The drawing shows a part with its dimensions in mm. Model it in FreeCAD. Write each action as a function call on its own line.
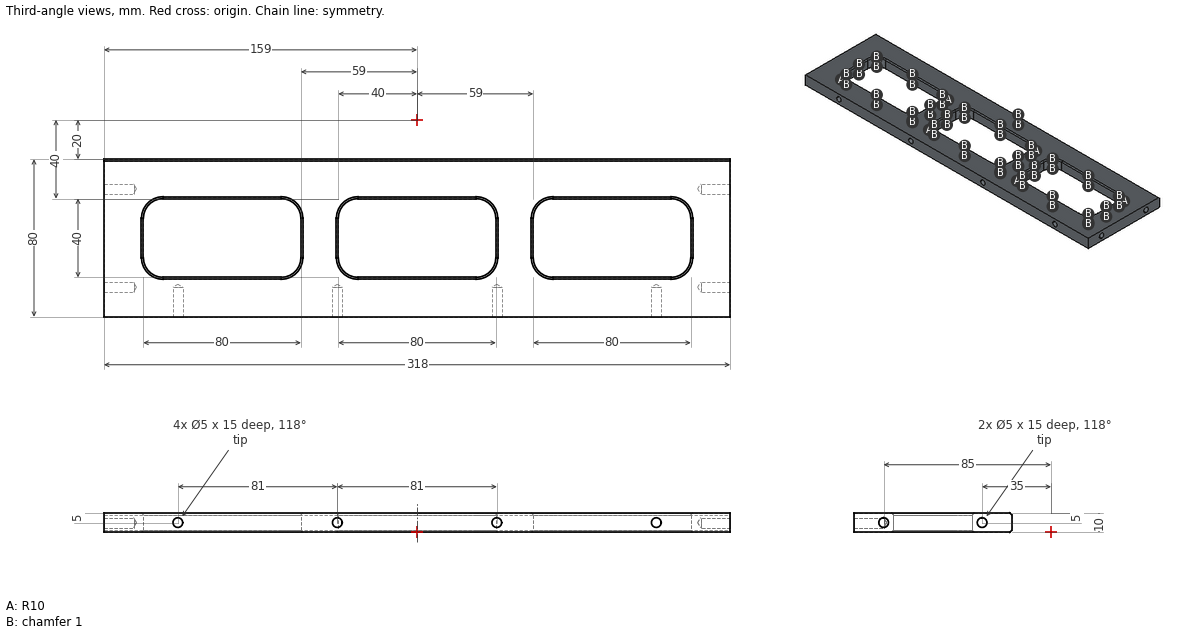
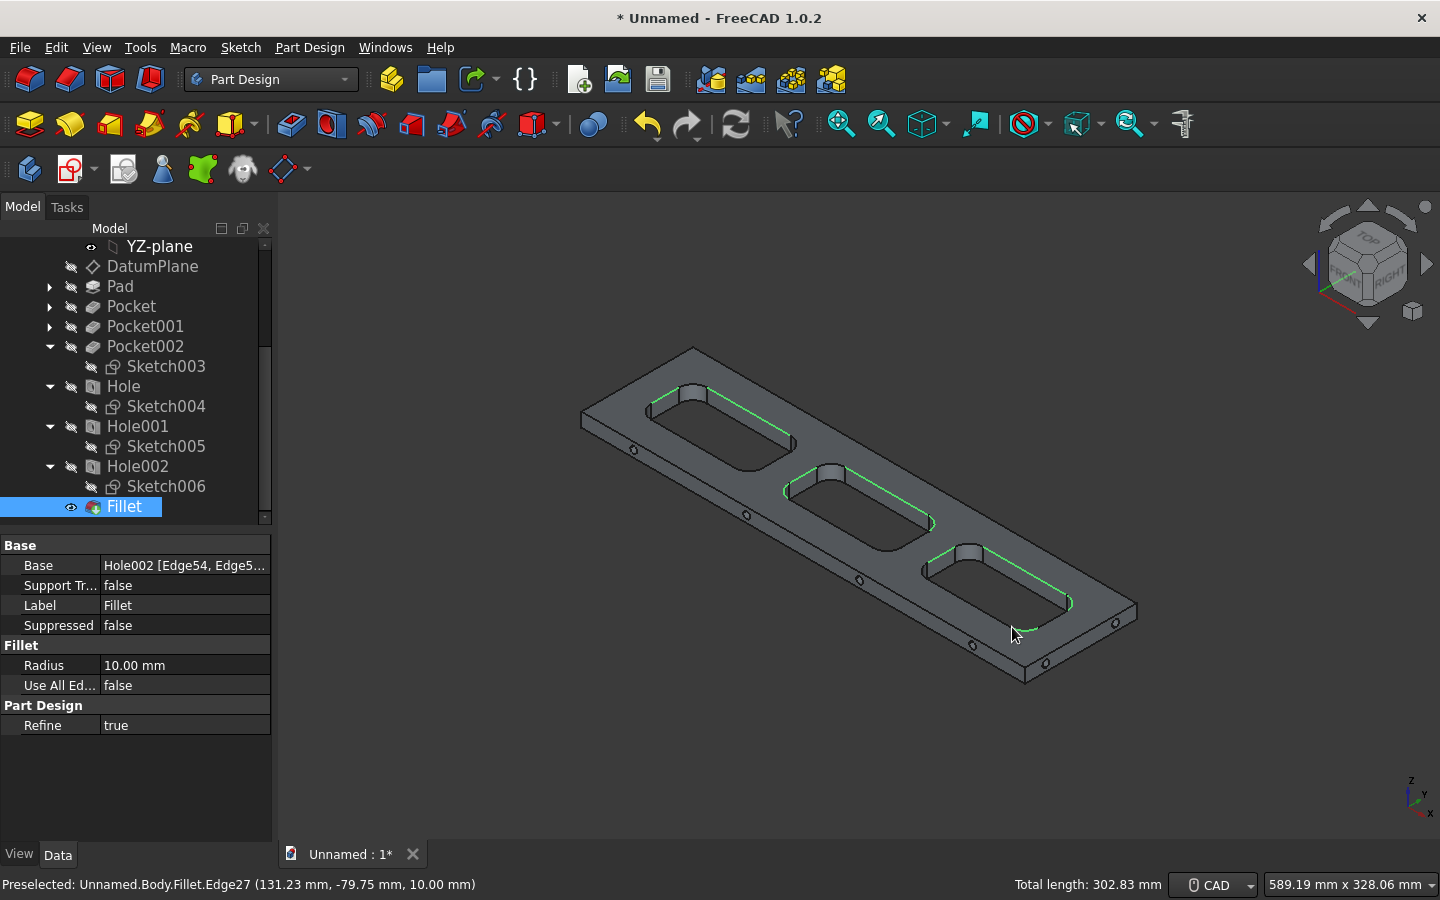
click(693, 383, ctrl)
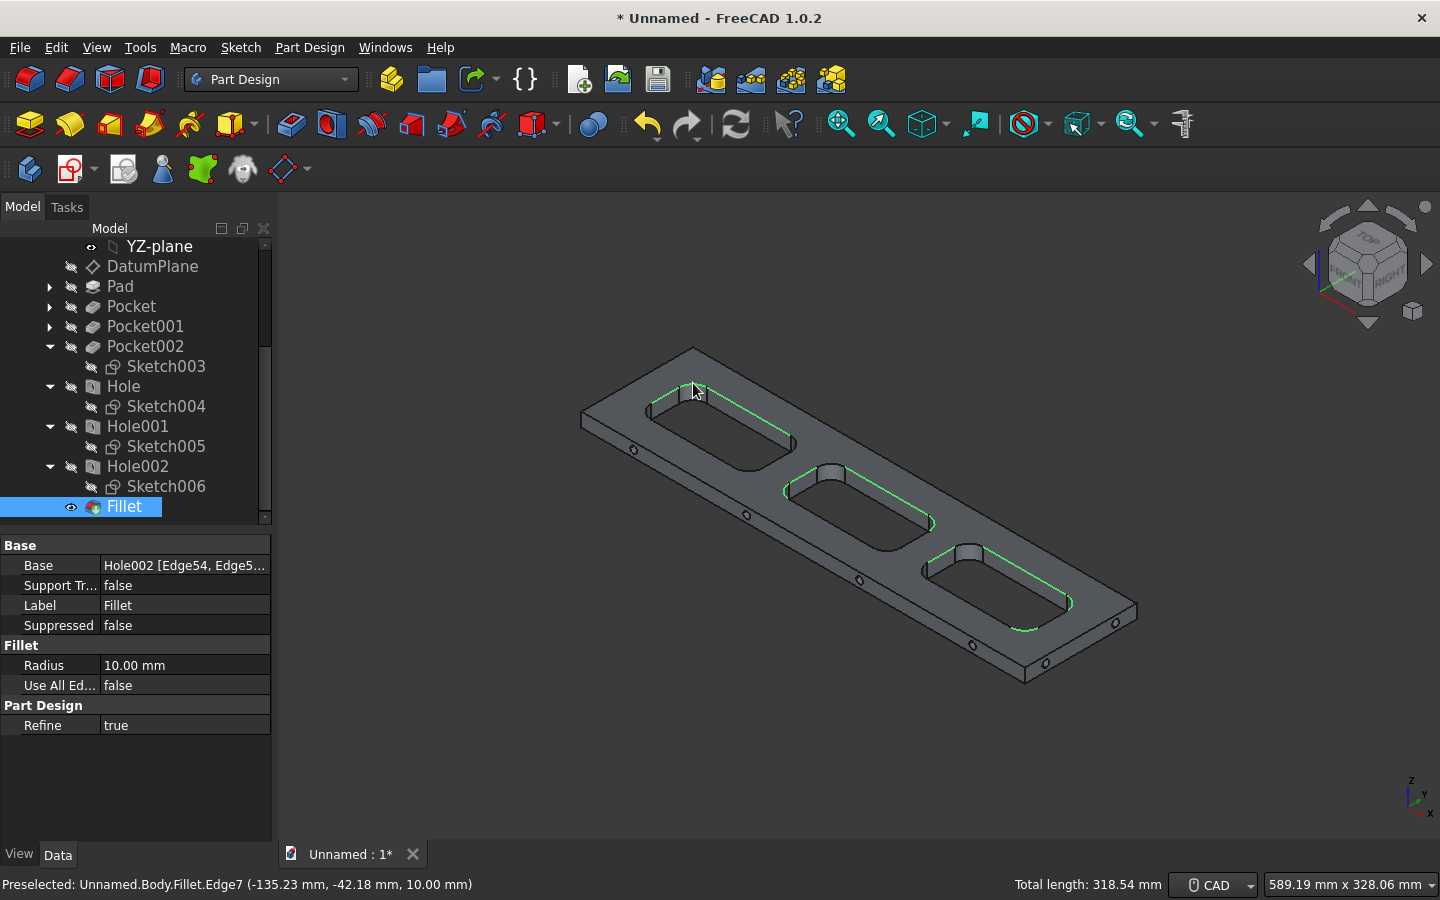
click(969, 543, ctrl)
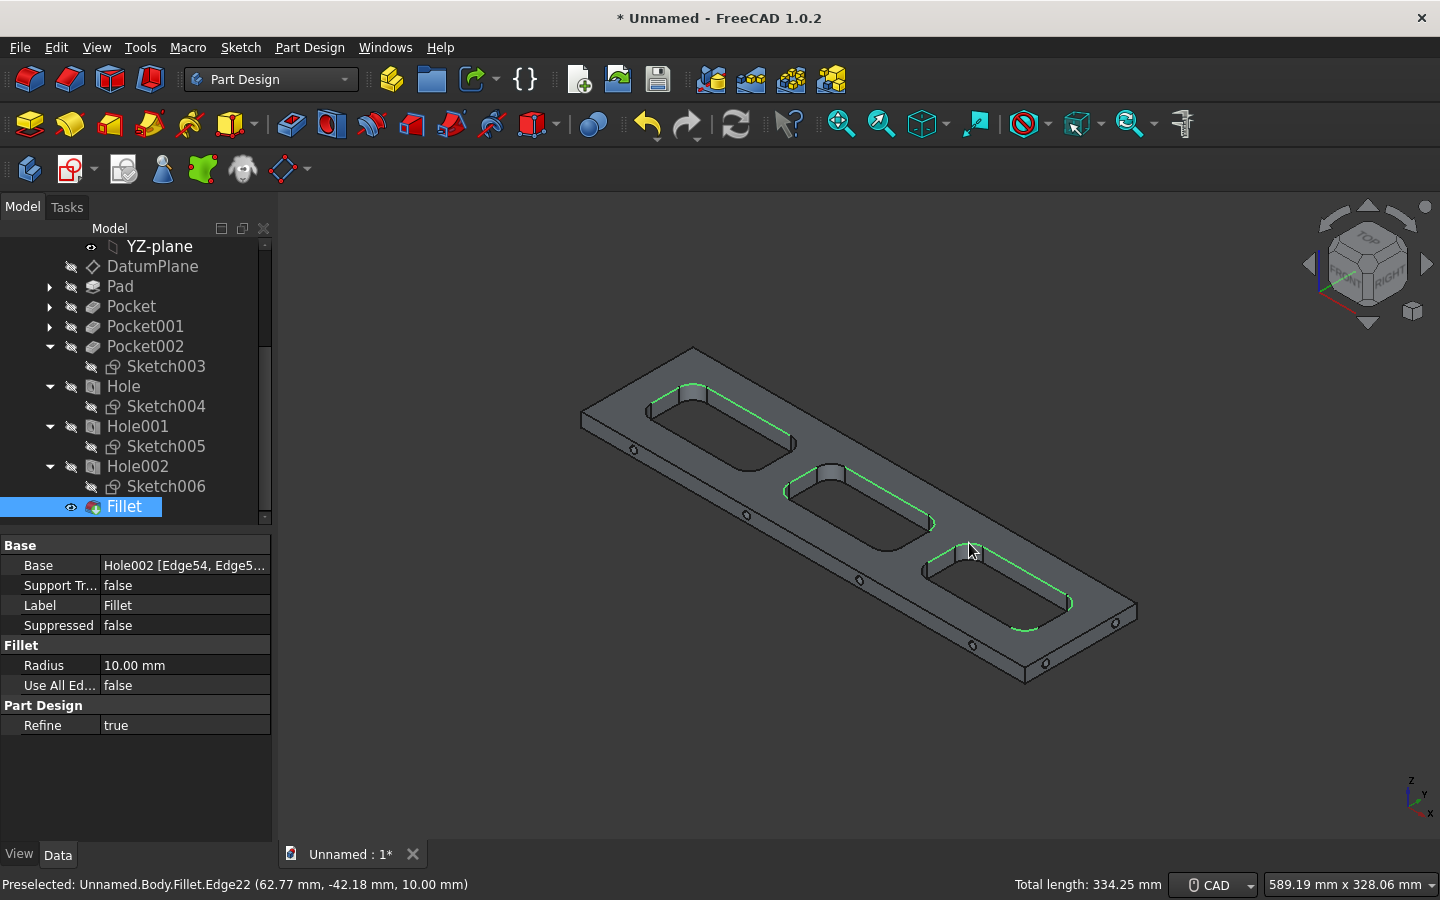
click(874, 547, ctrl)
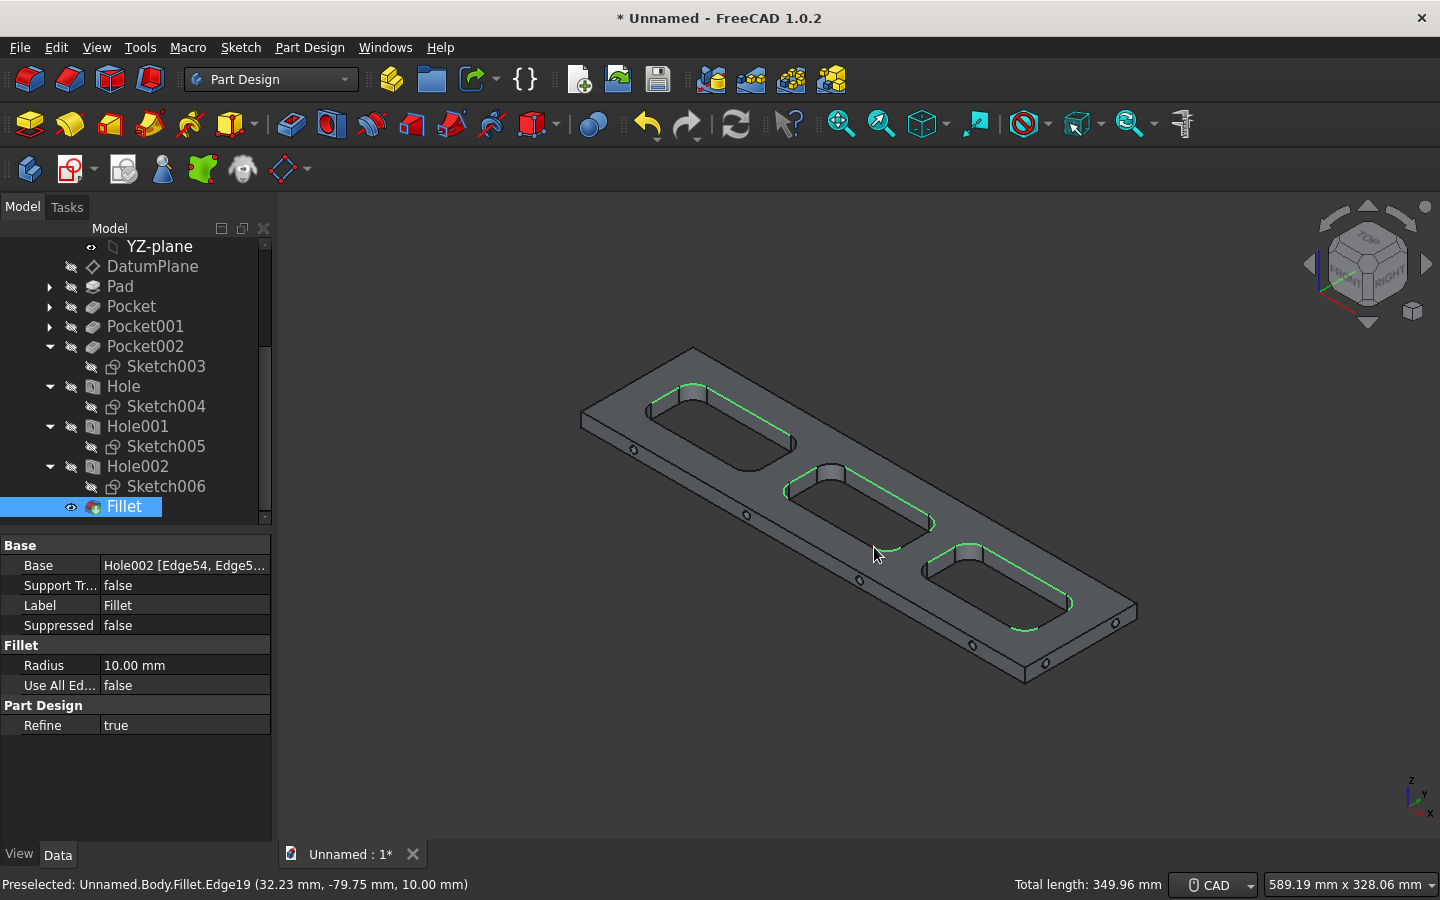
click(796, 443, ctrl)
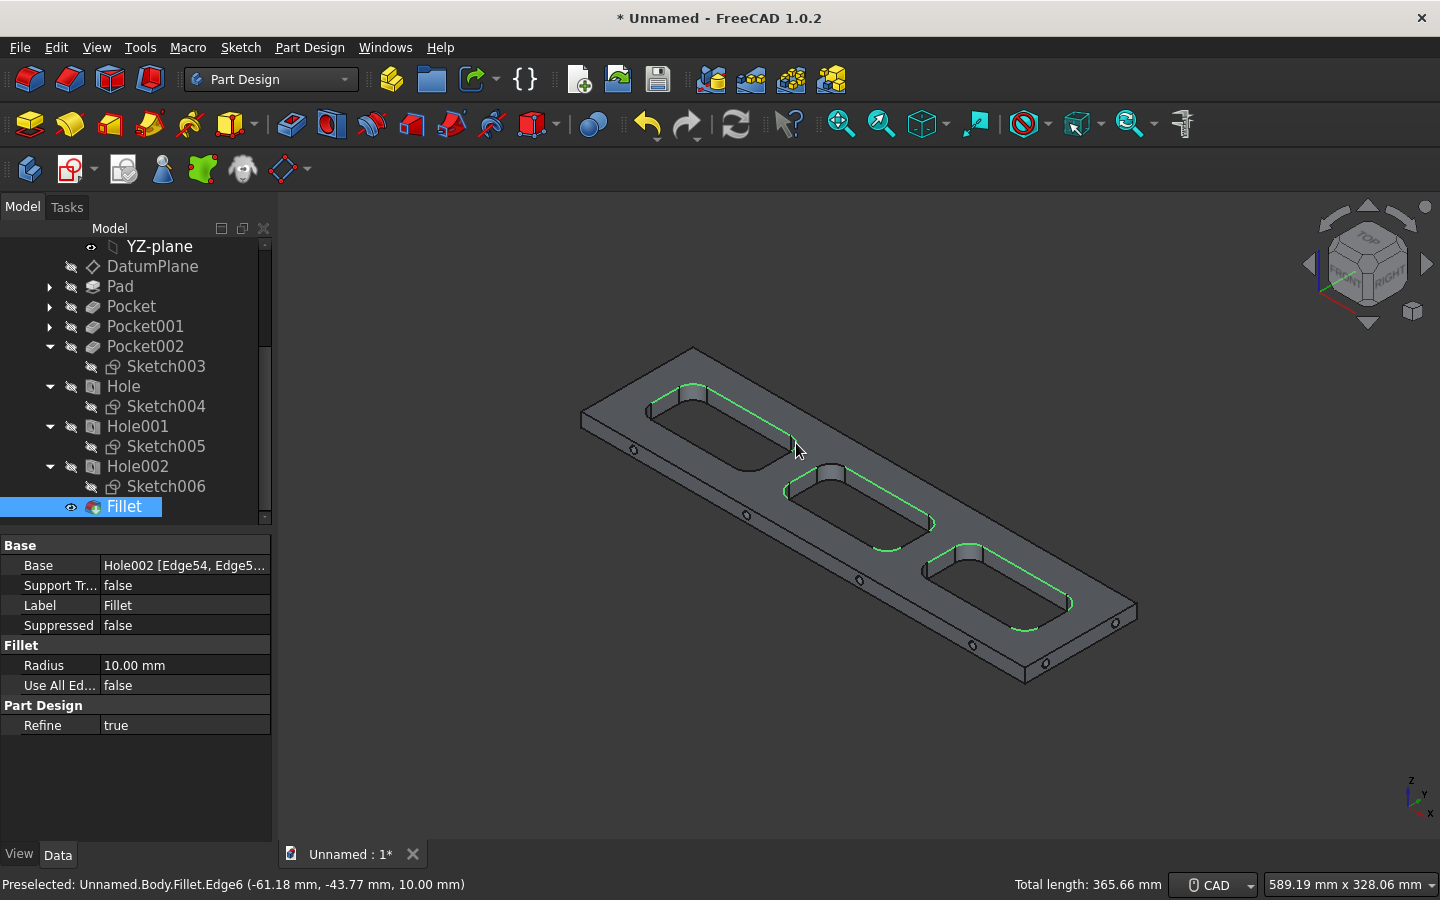
click(831, 463, ctrl)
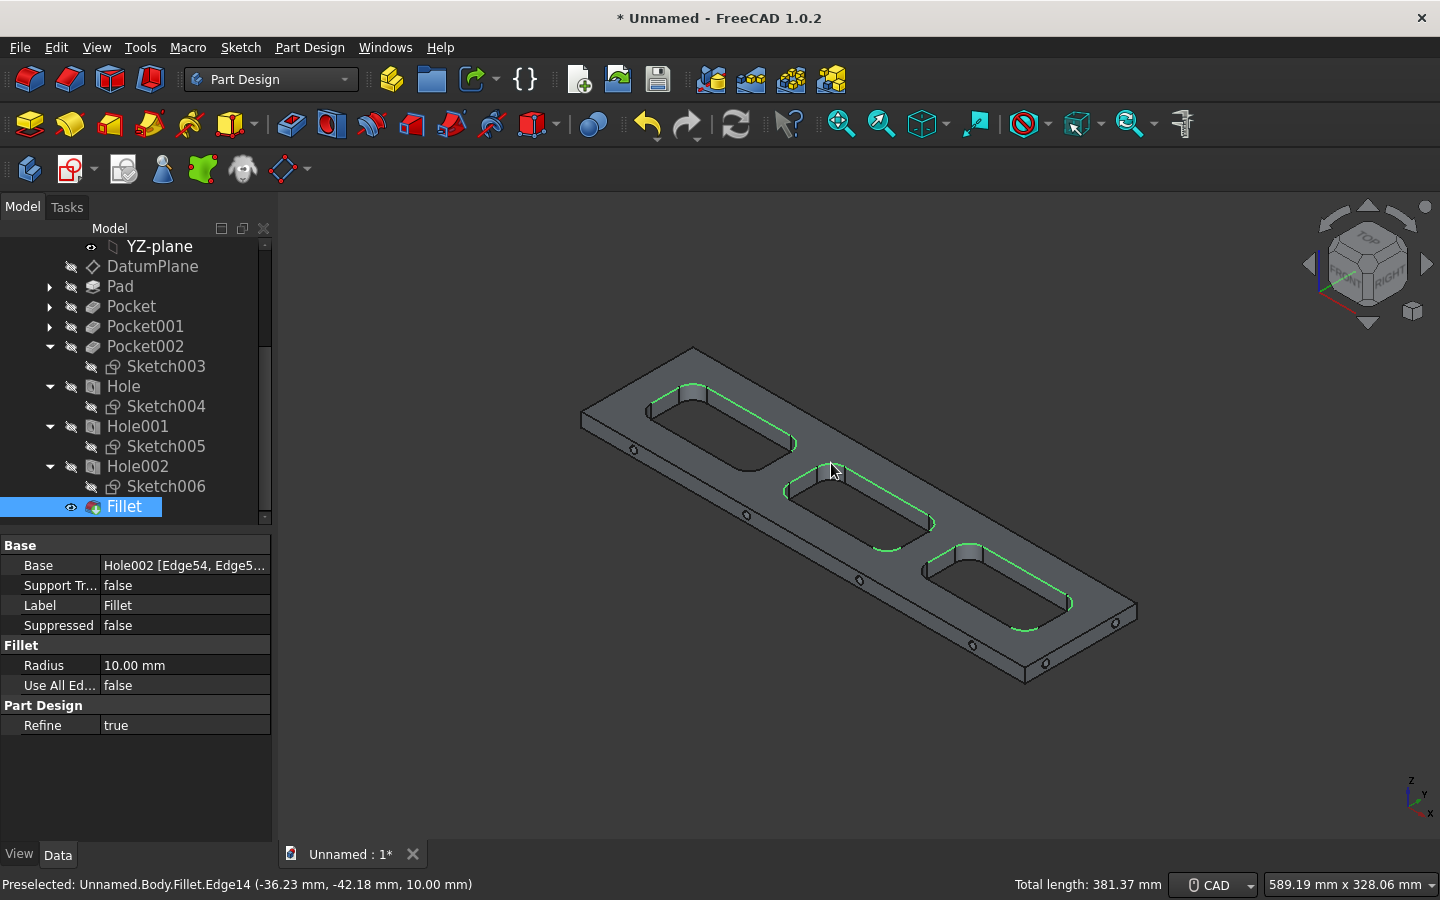
click(837, 480, ctrl)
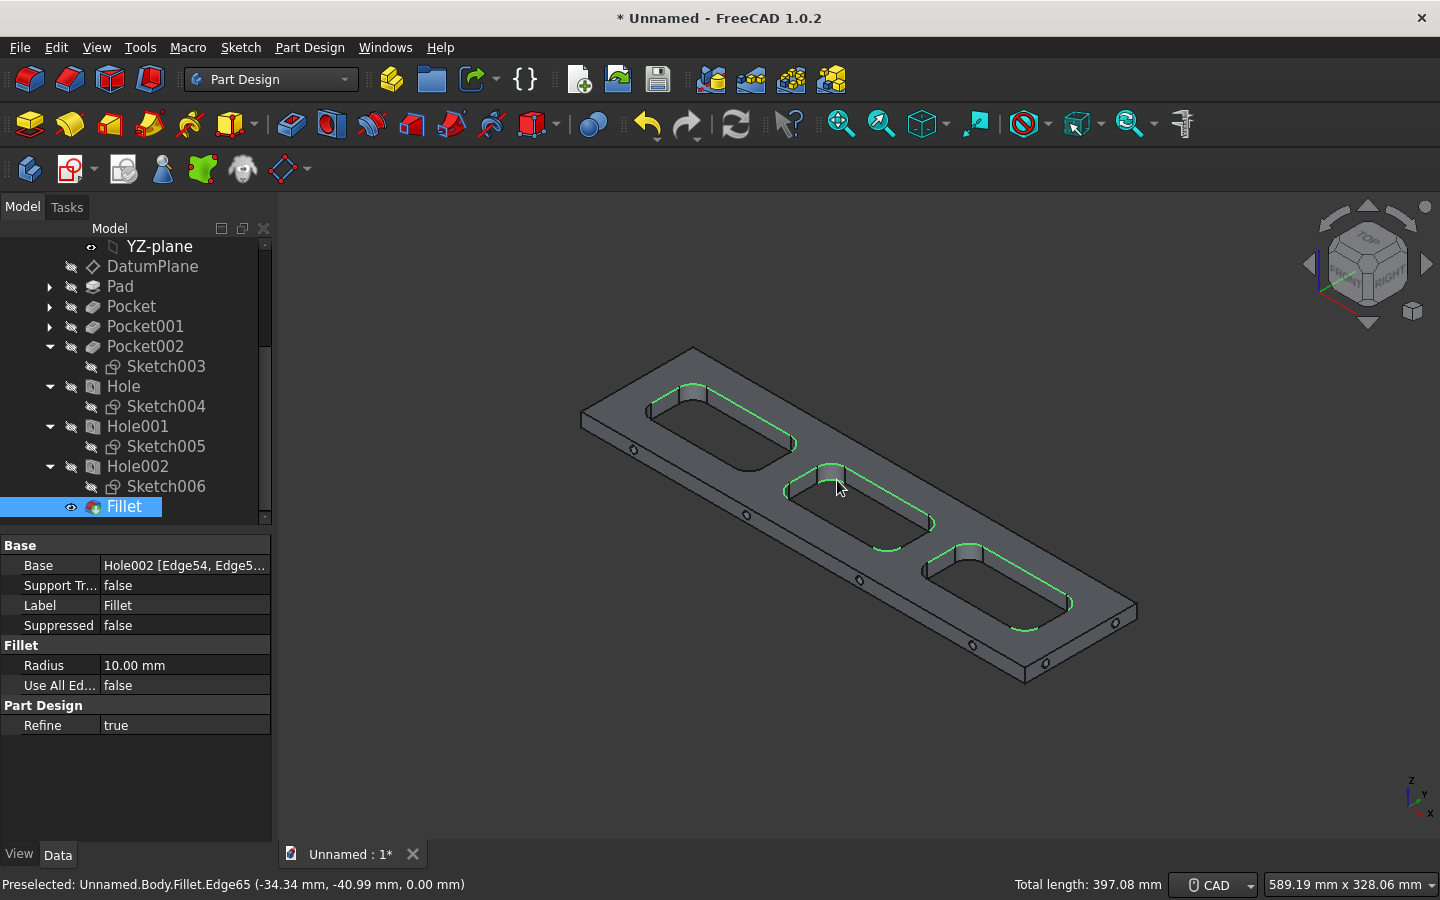
click(736, 467, ctrl)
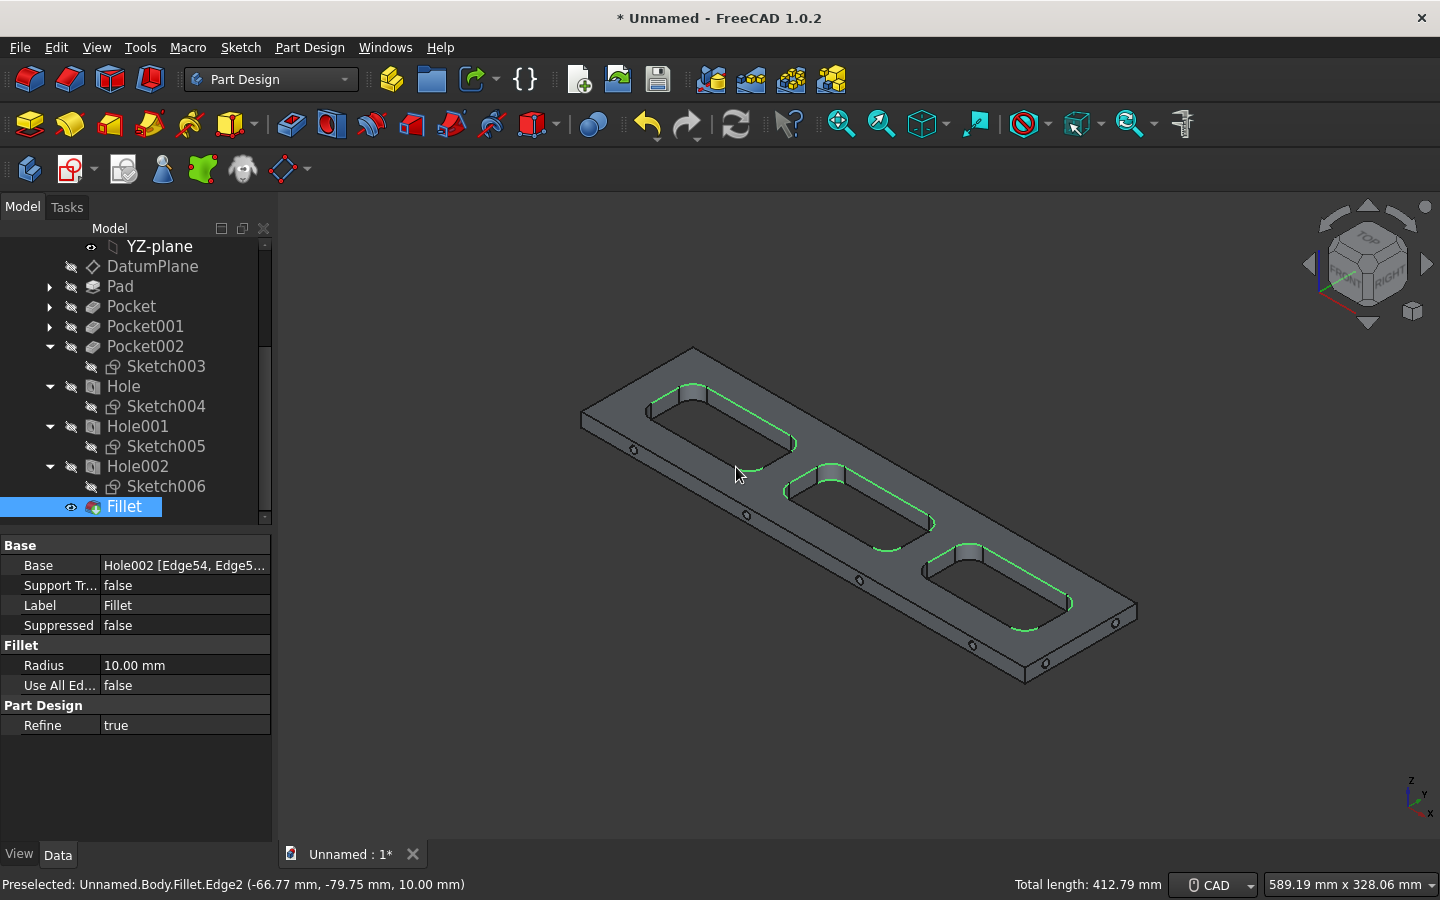
click(646, 412, ctrl)